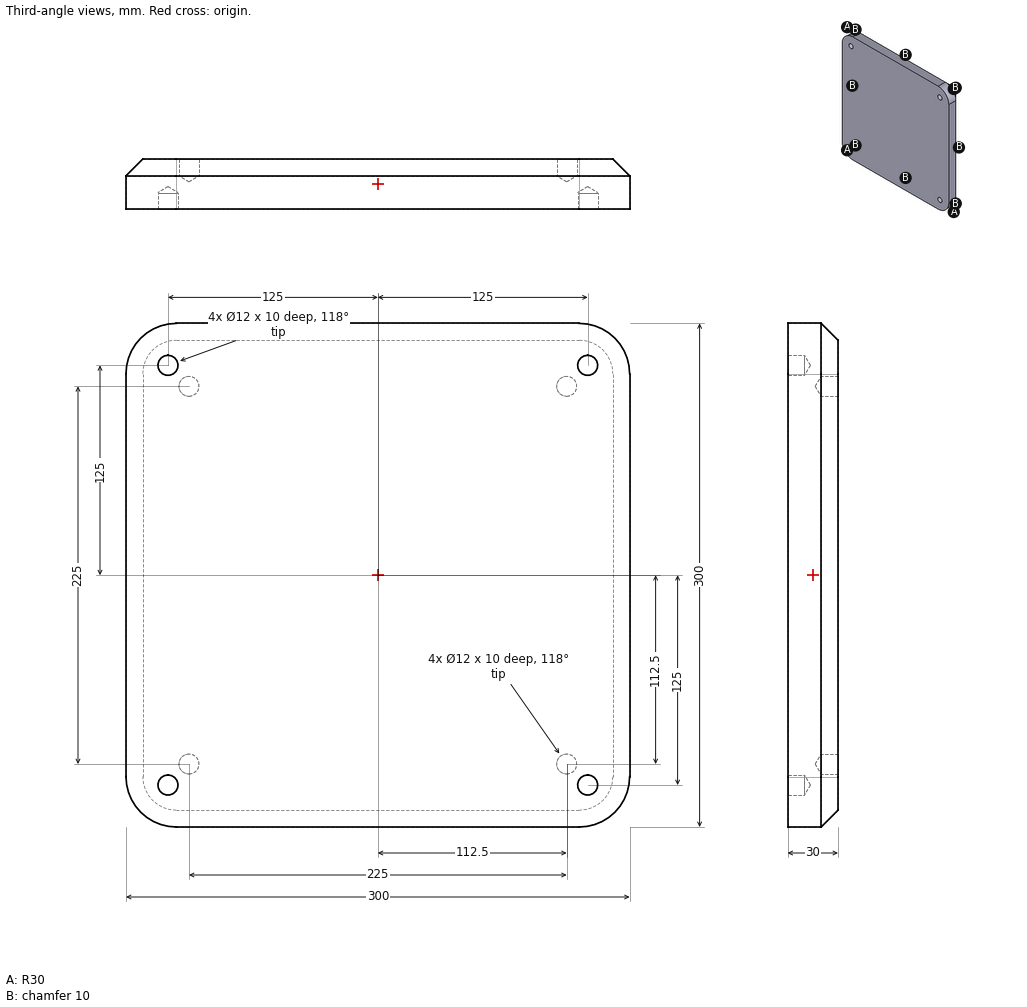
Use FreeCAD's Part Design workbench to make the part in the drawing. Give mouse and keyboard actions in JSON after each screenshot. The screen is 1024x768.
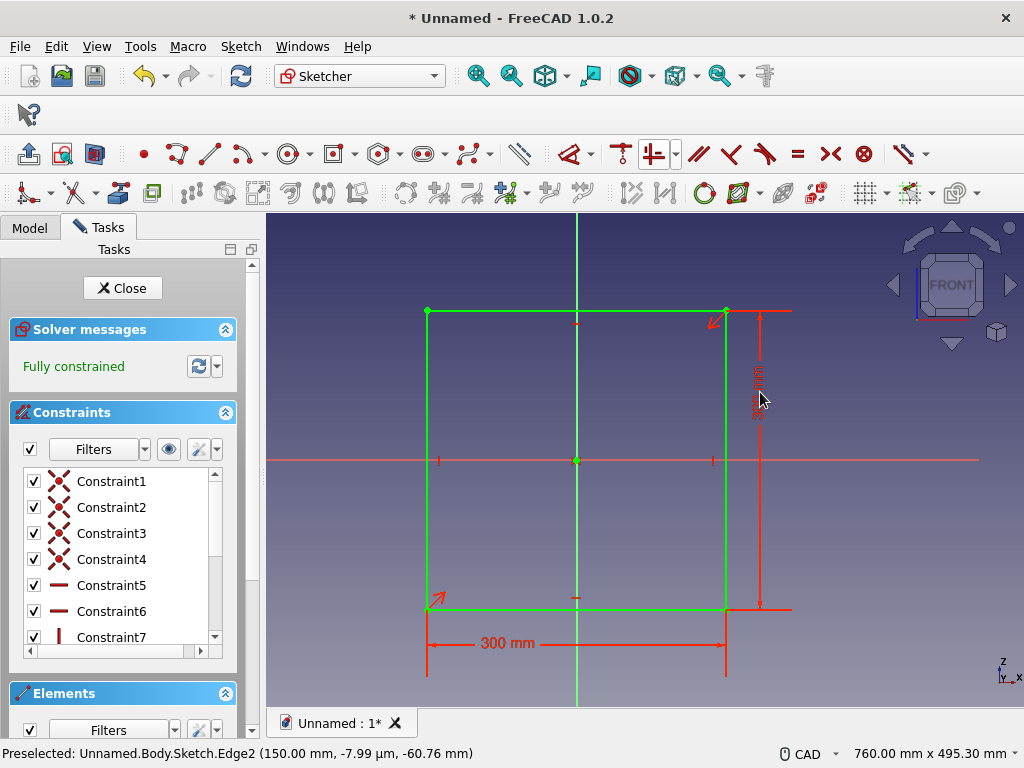
{"action": "left_click", "coordinate": [123, 288]}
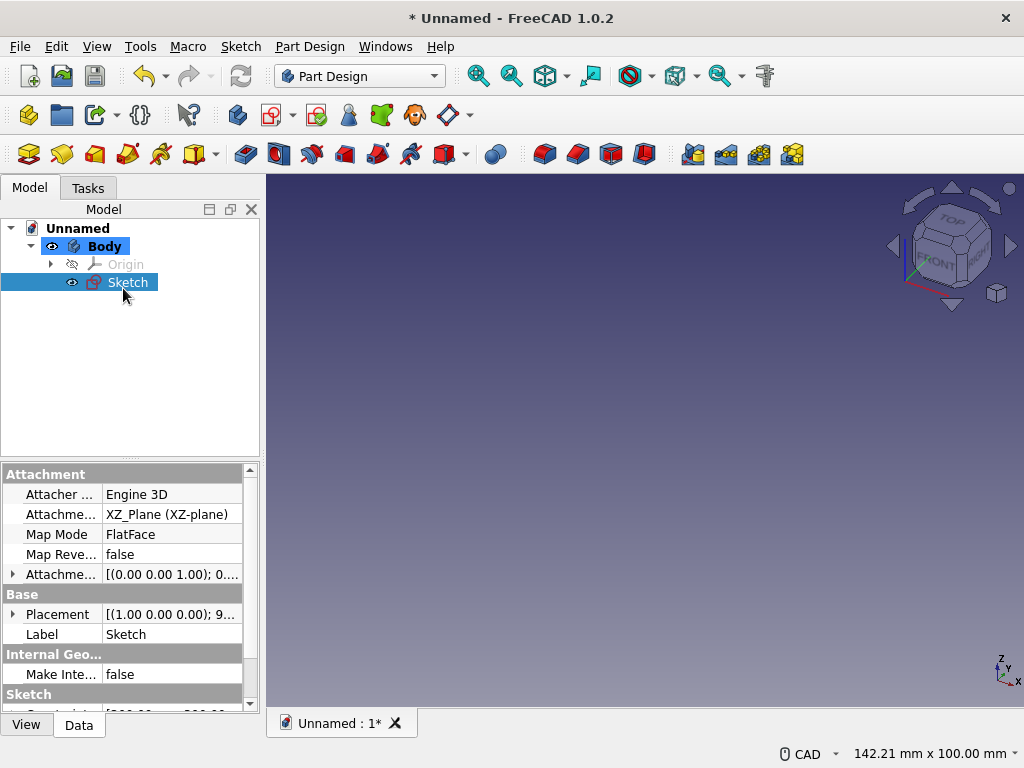
{"action": "left_click", "coordinate": [29, 154]}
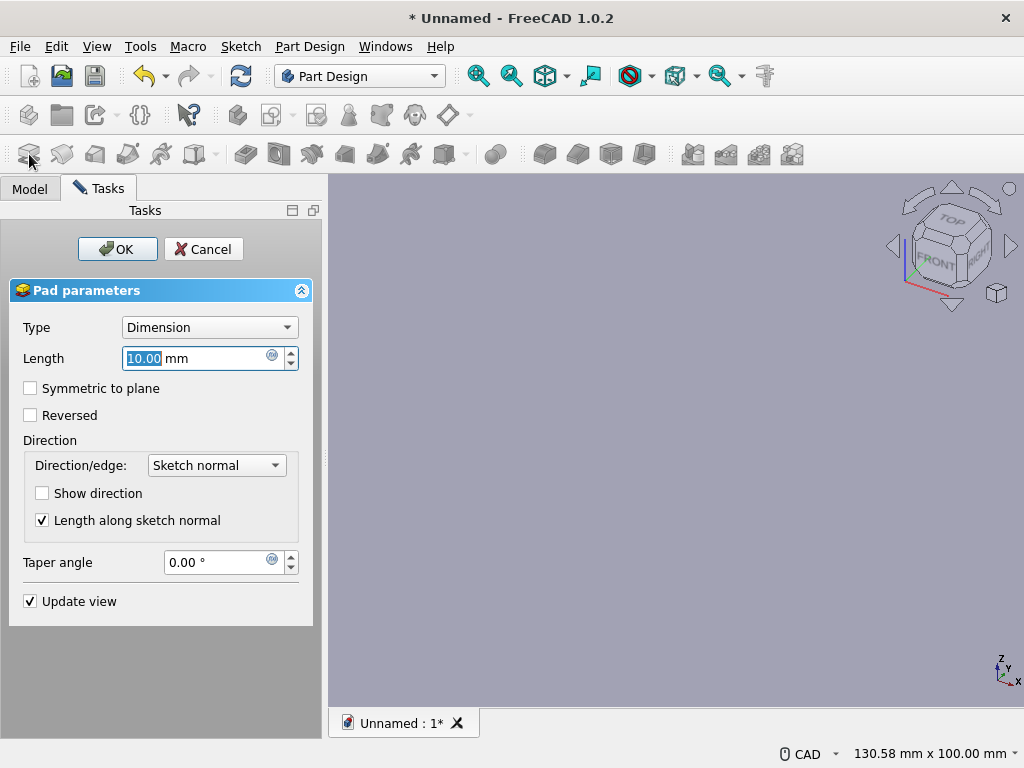
{"action": "type", "text": "30"}
{"action": "key", "text": "Tab"}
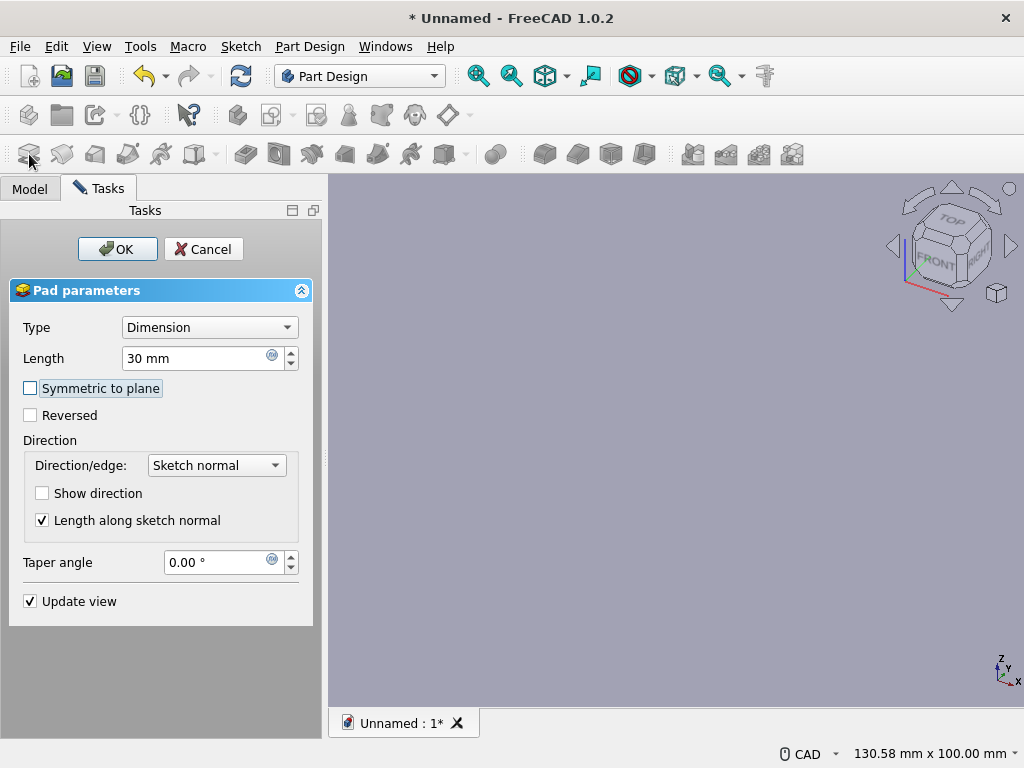
{"action": "left_click", "coordinate": [31, 388]}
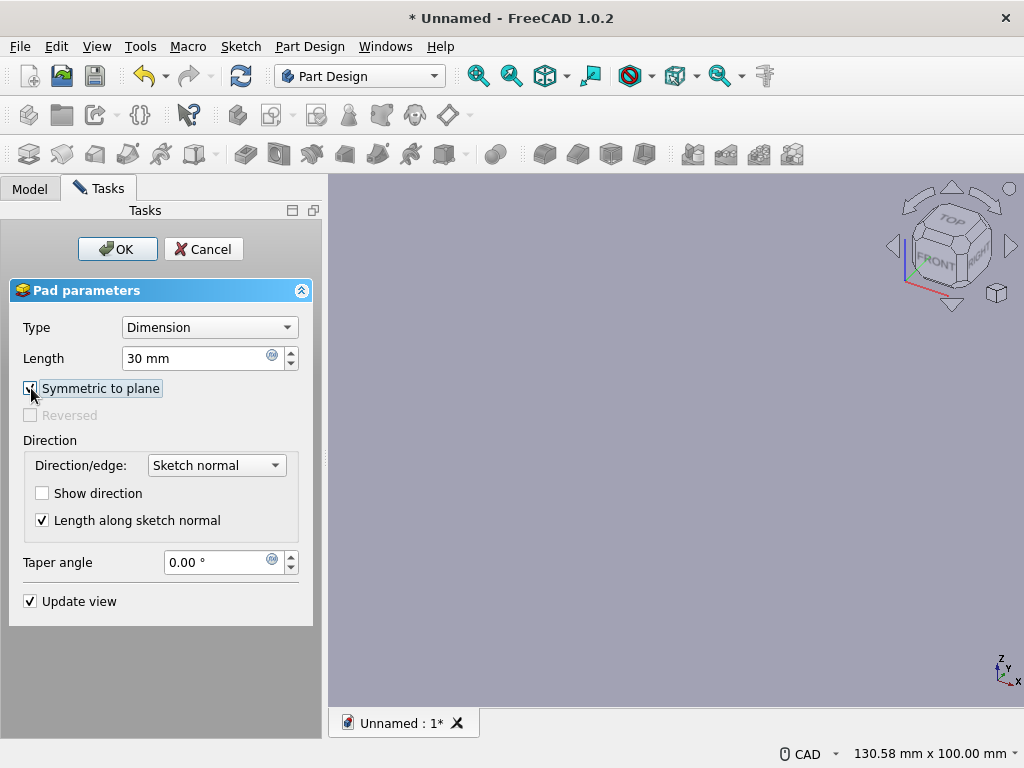
{"action": "left_click", "coordinate": [118, 249]}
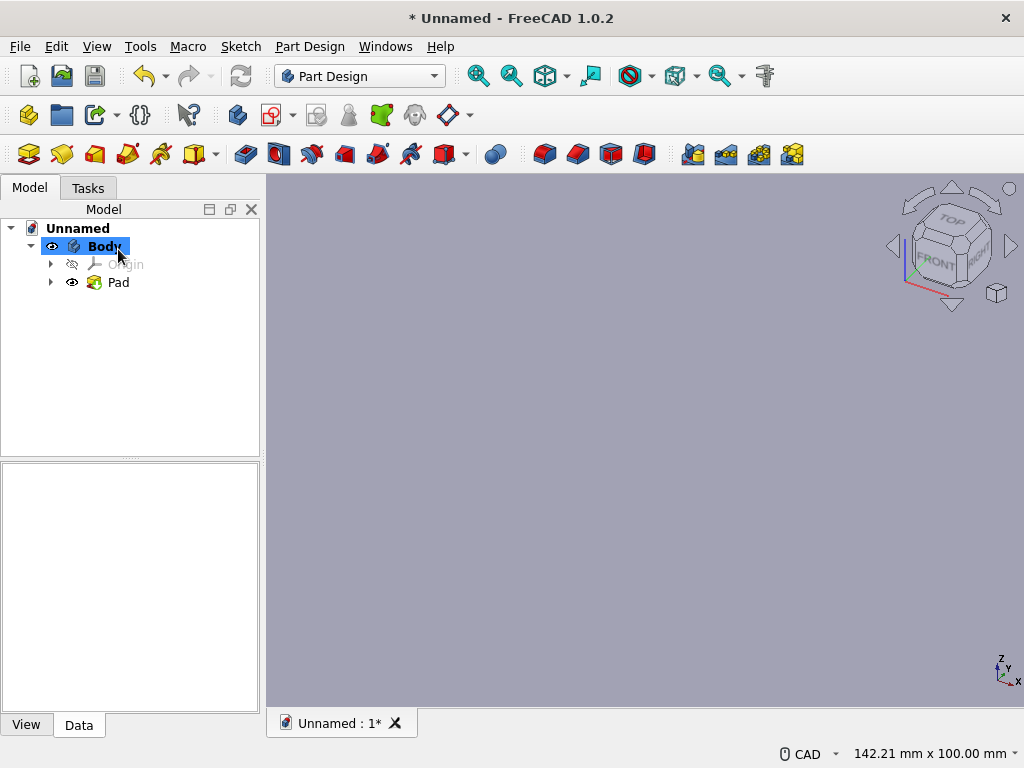
{"action": "left_click", "coordinate": [479, 76]}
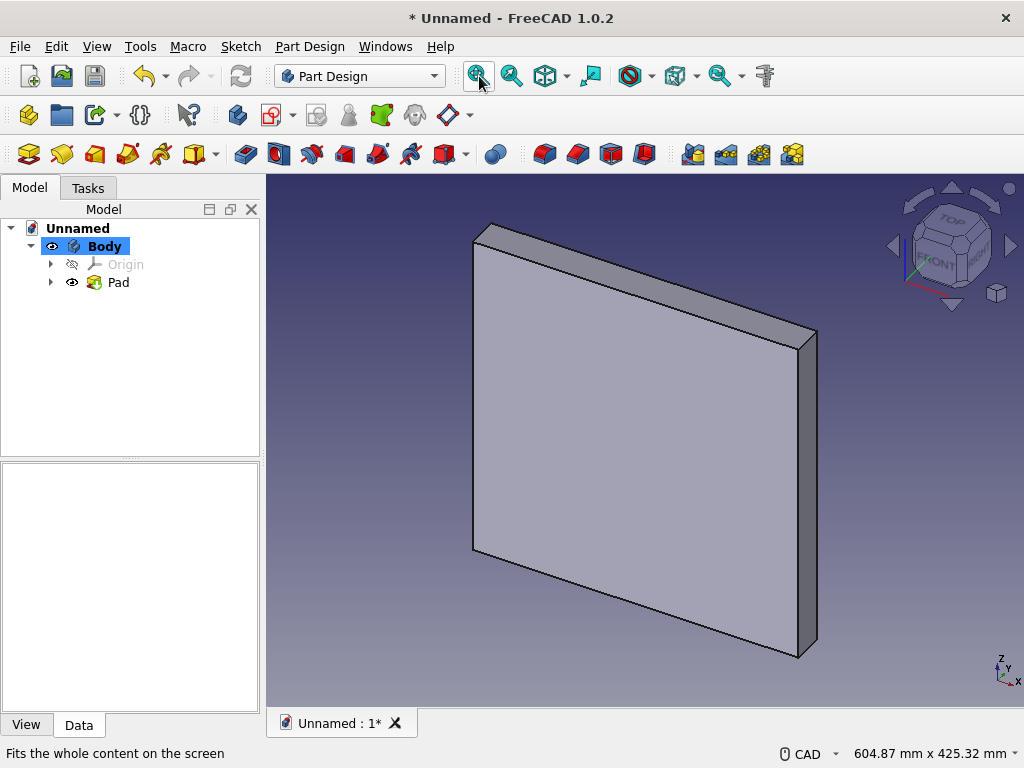
{"action": "left_click", "coordinate": [808, 339]}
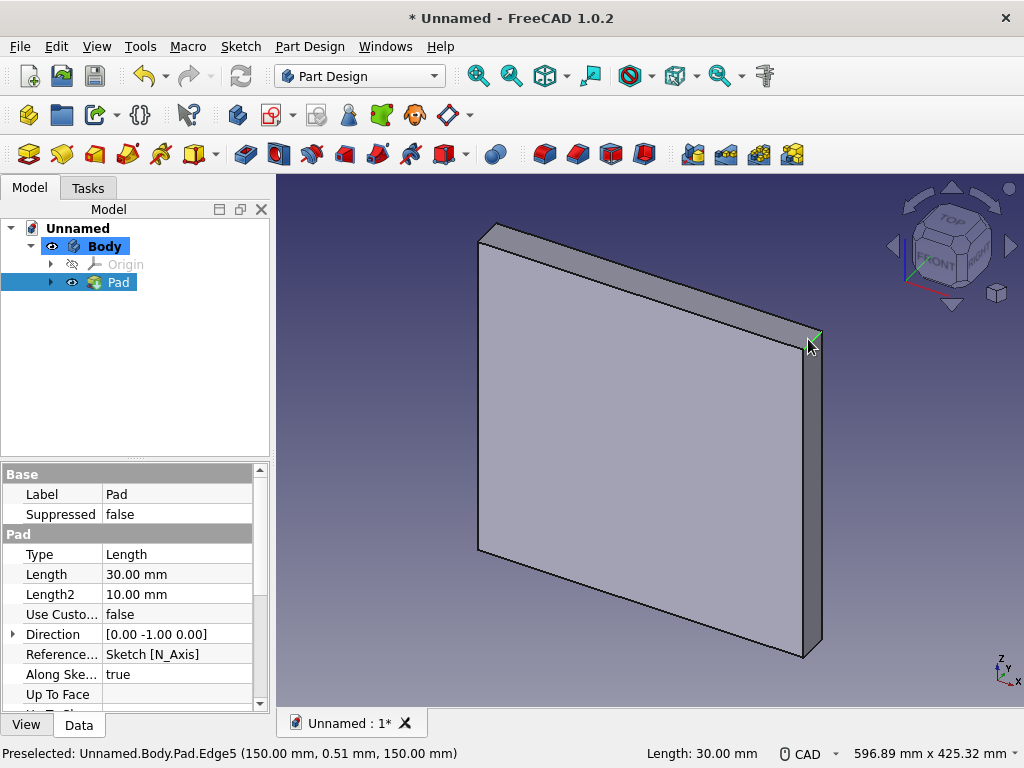
{"action": "key", "text": "0"}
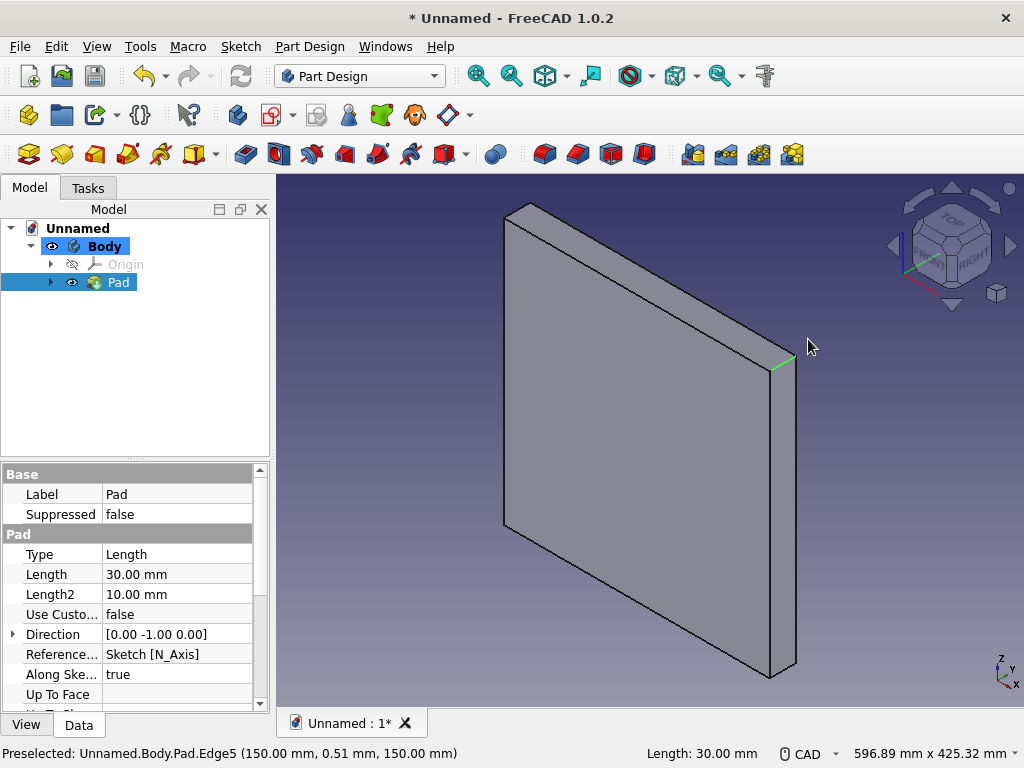
{"action": "key", "text": "2"}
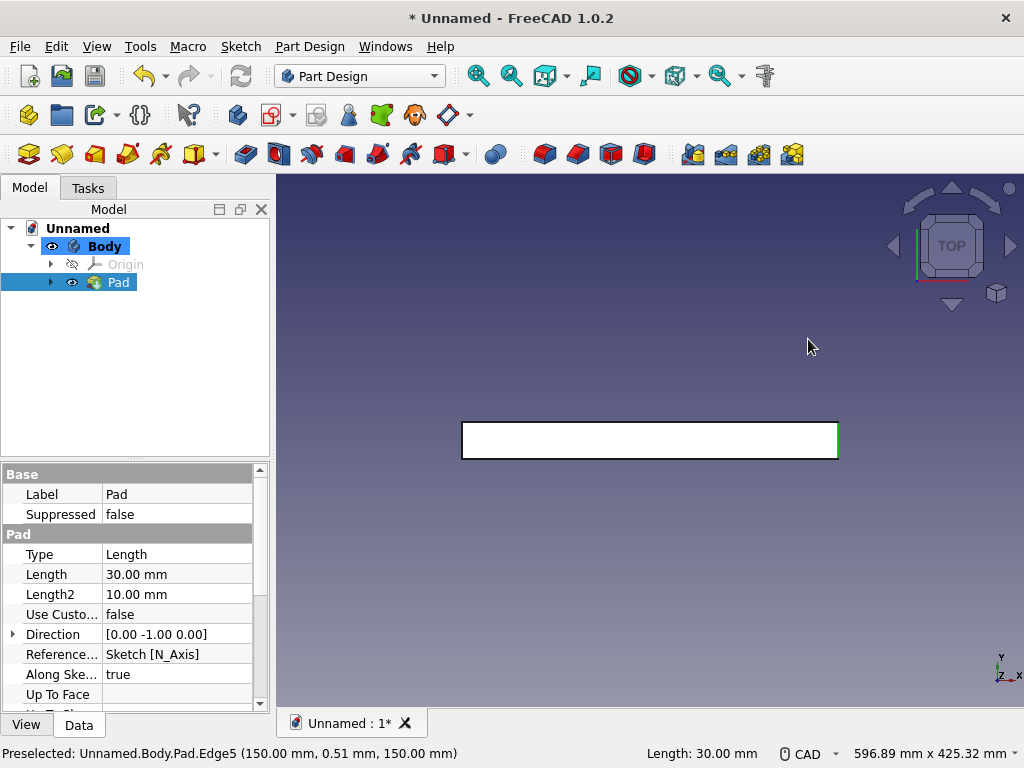
{"action": "left_click", "coordinate": [462, 440], "text": "ctrl"}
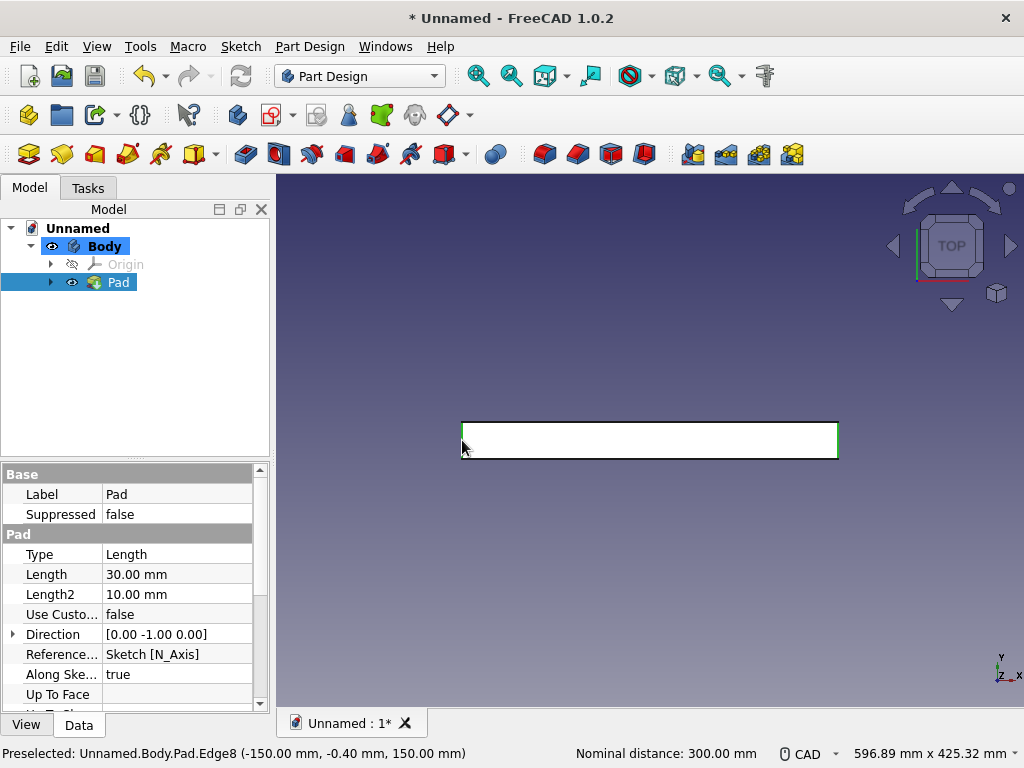
{"action": "key", "text": "1"}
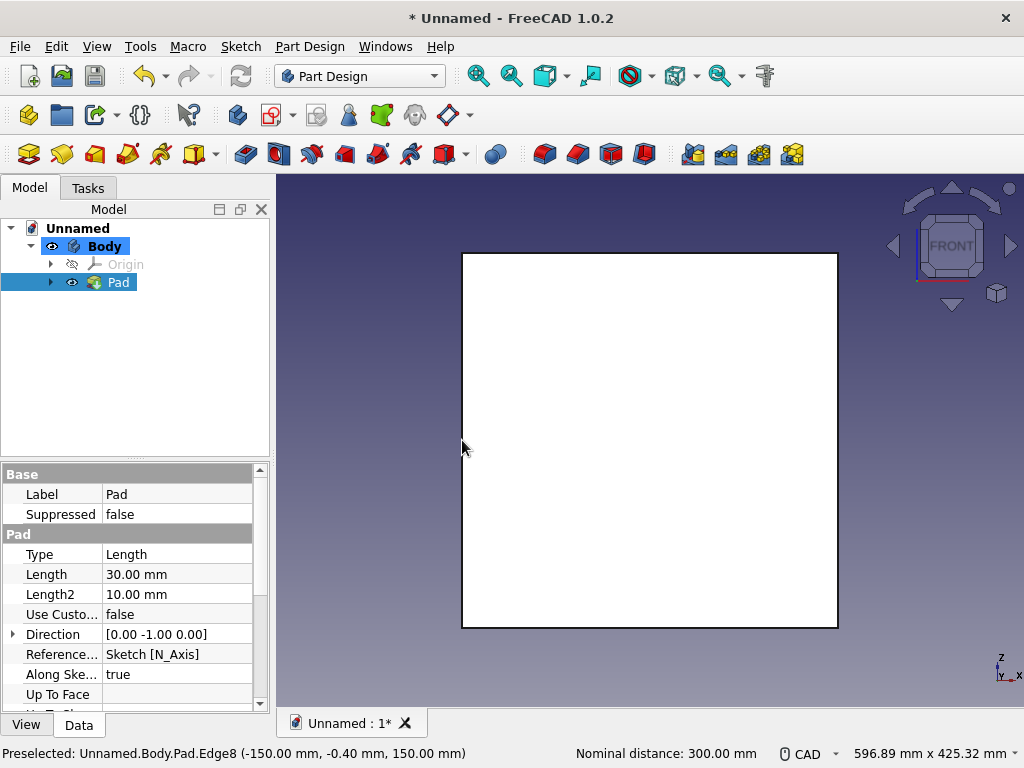
{"action": "key", "text": "3"}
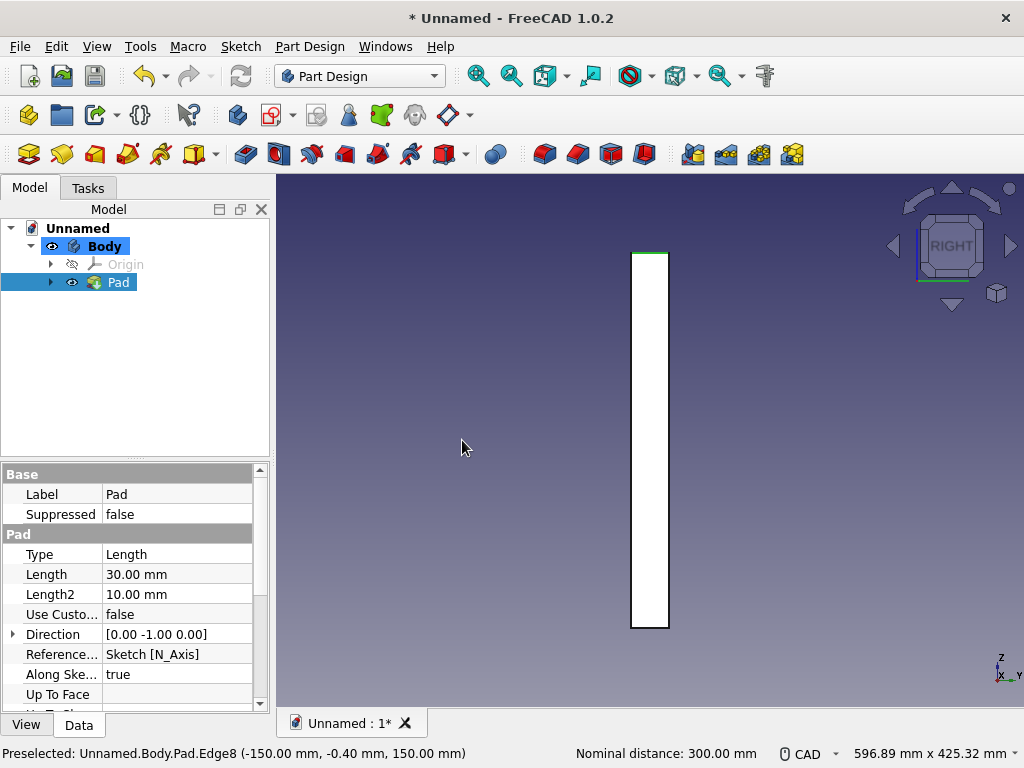
{"action": "left_click", "coordinate": [650, 627], "text": "ctrl"}